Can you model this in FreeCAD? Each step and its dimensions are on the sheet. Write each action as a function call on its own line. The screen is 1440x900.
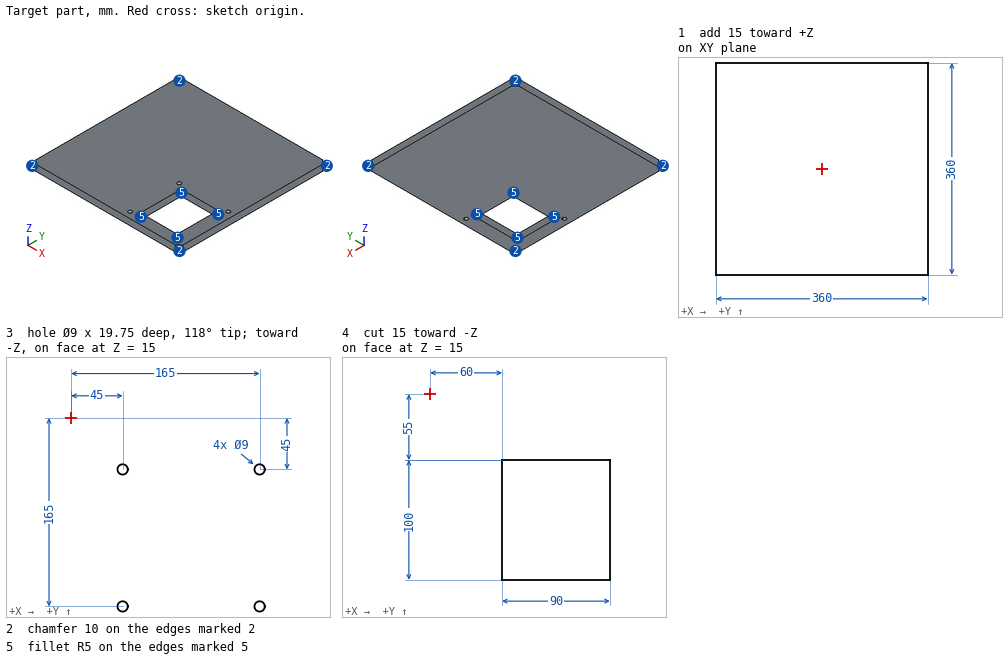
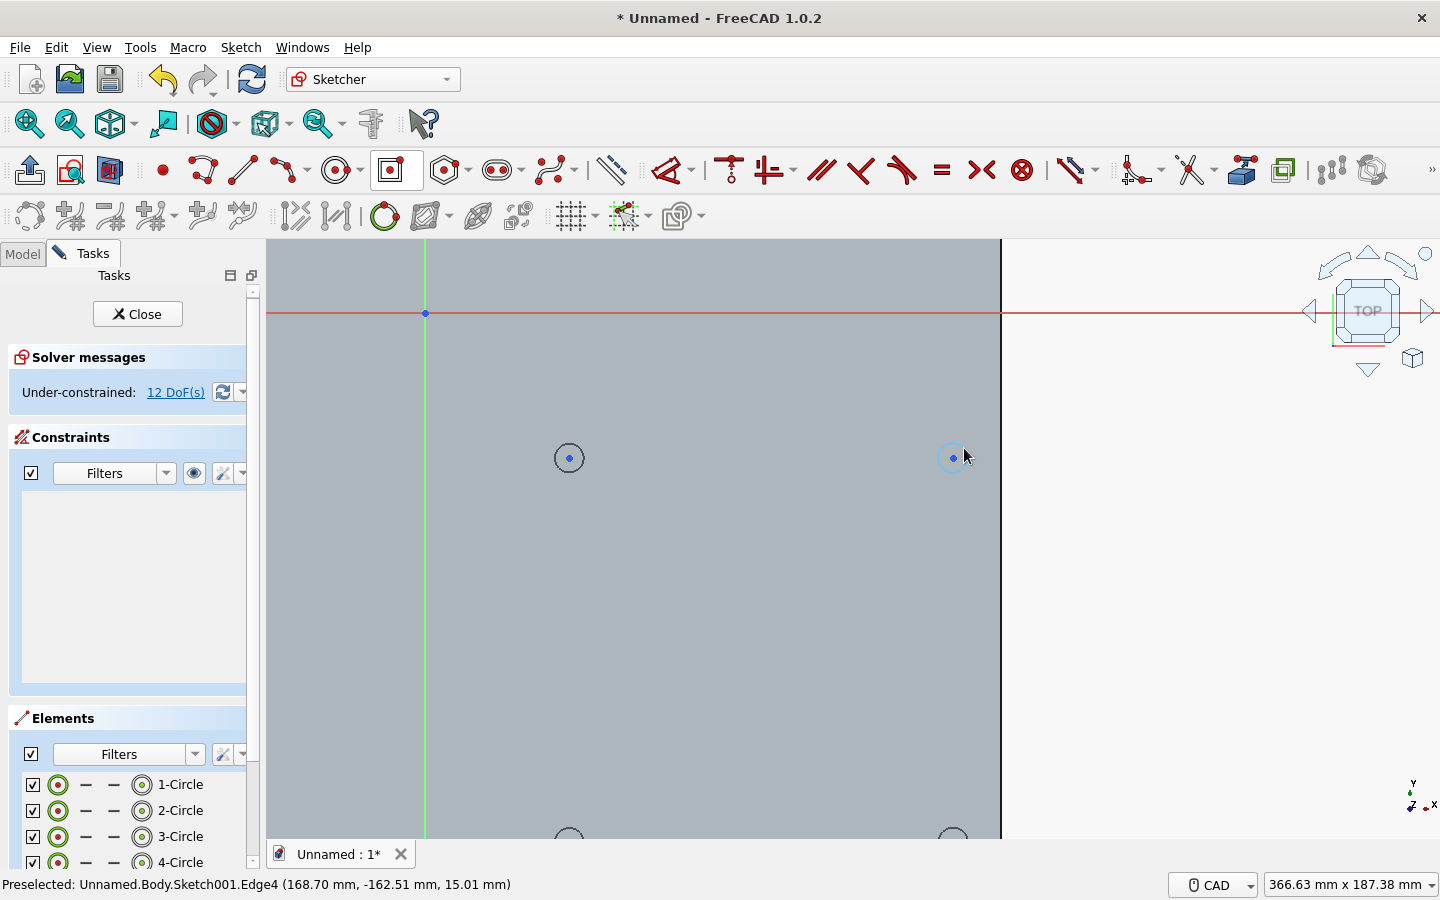
click(964, 448)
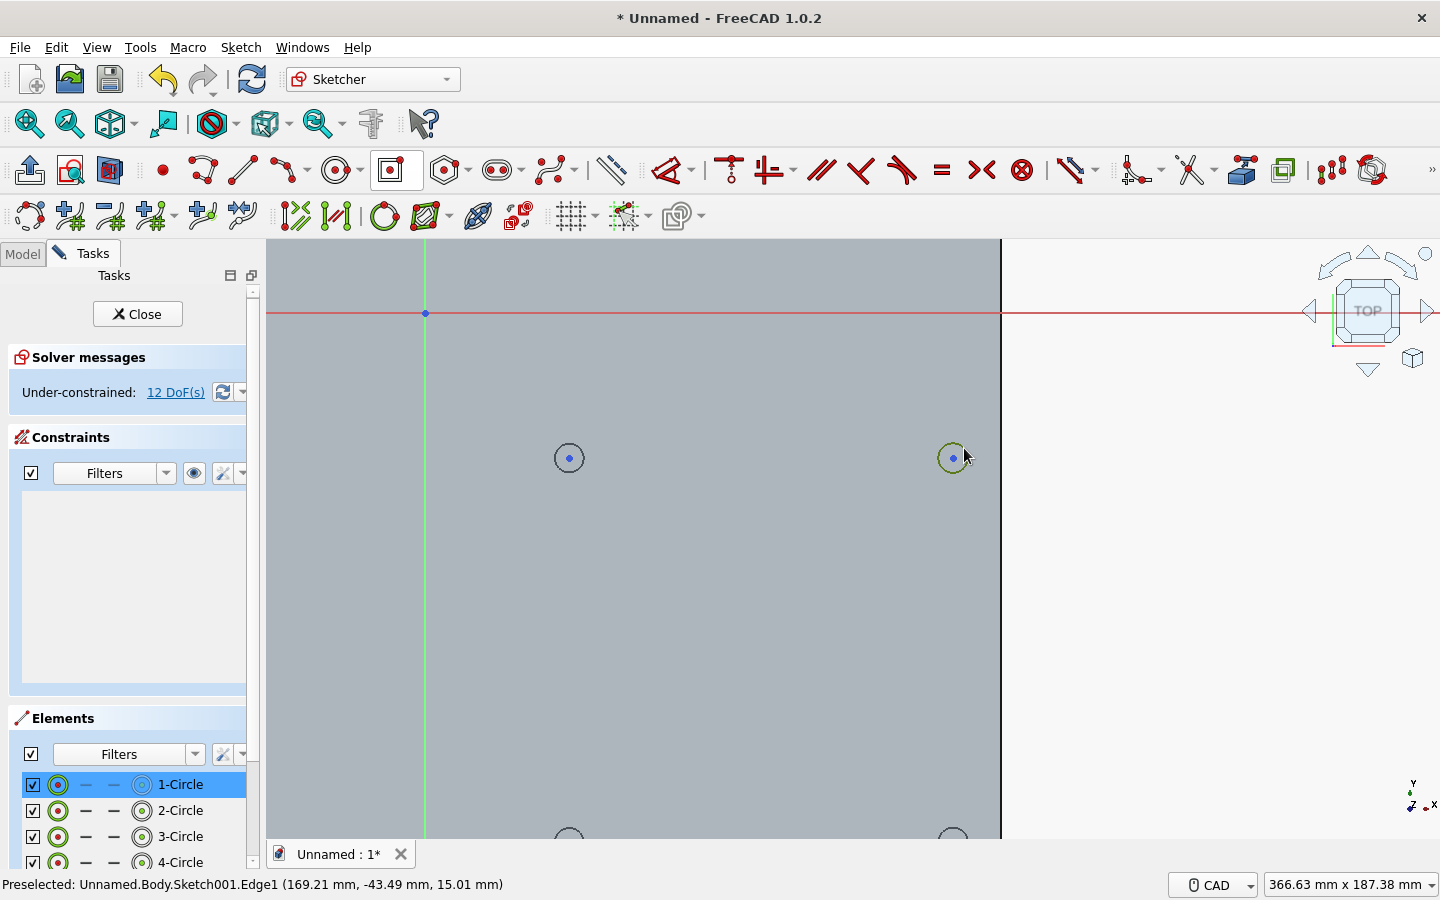
click(579, 448)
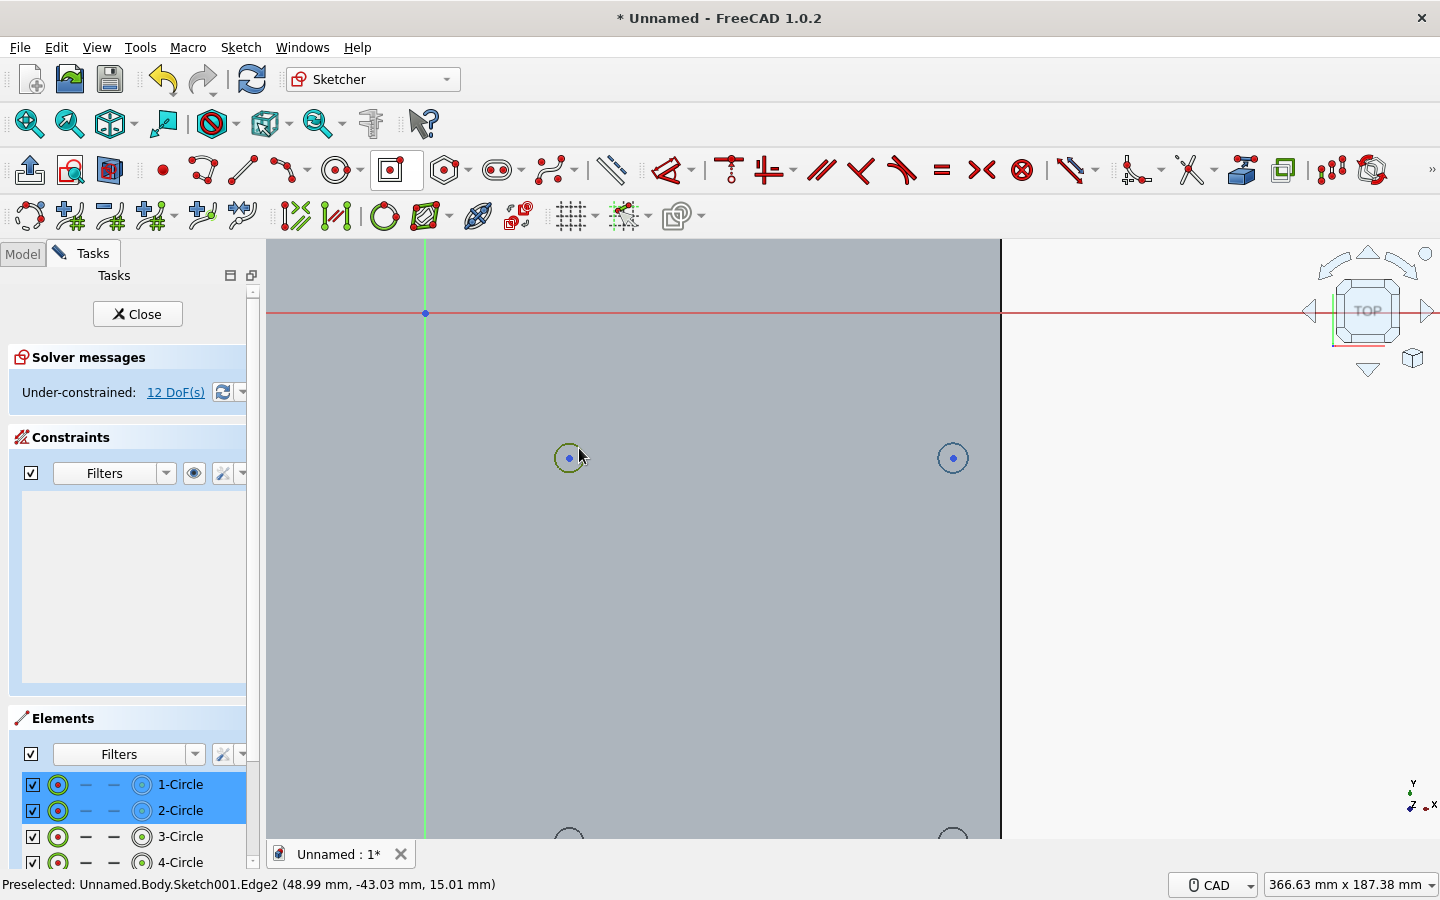
scroll(964, 446, down, 2)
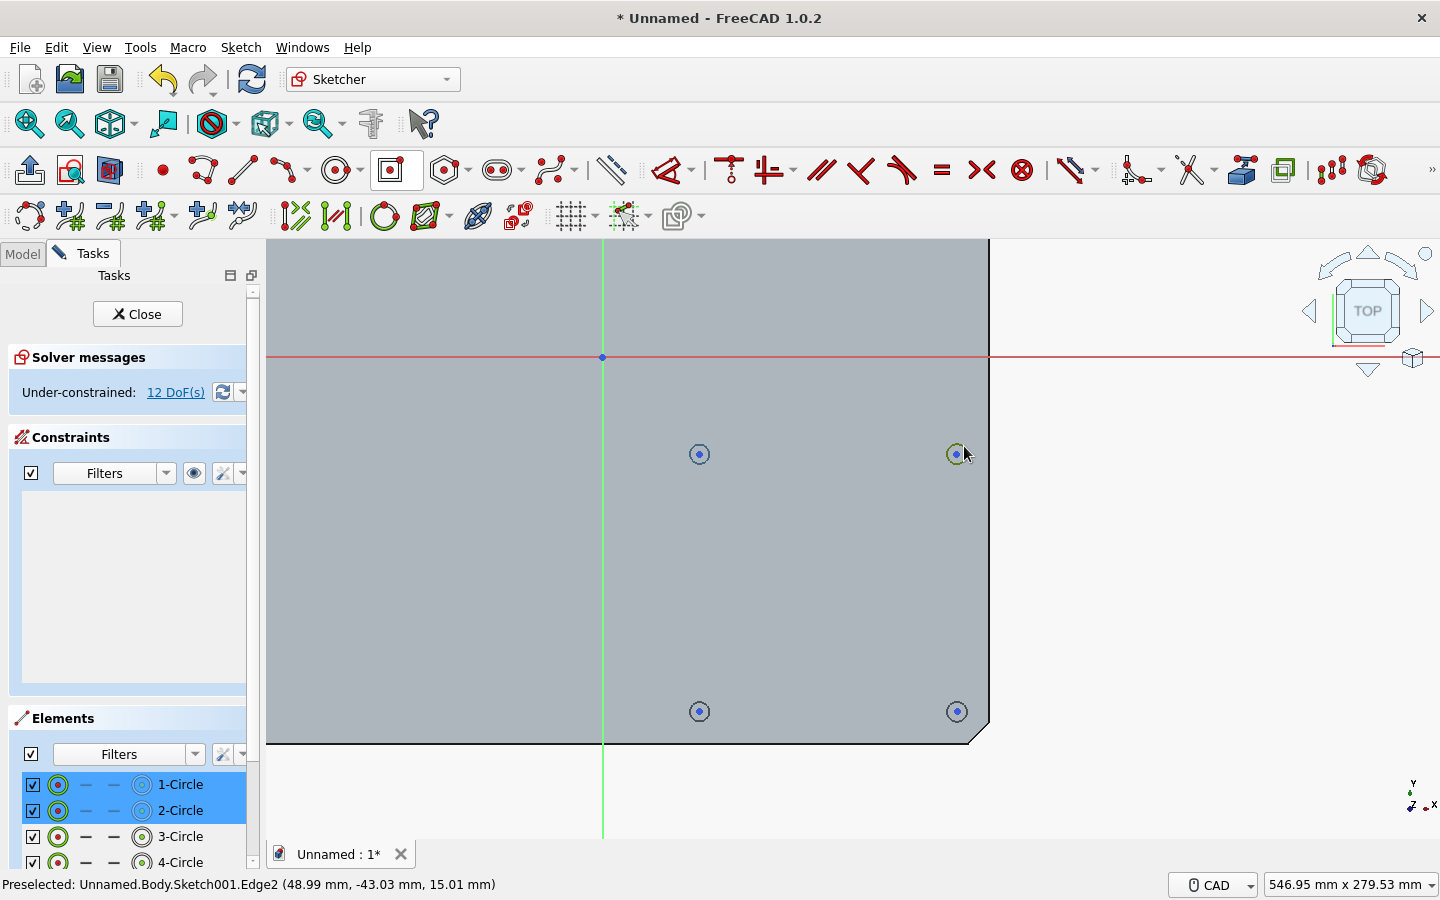
scroll(706, 705, up, 2)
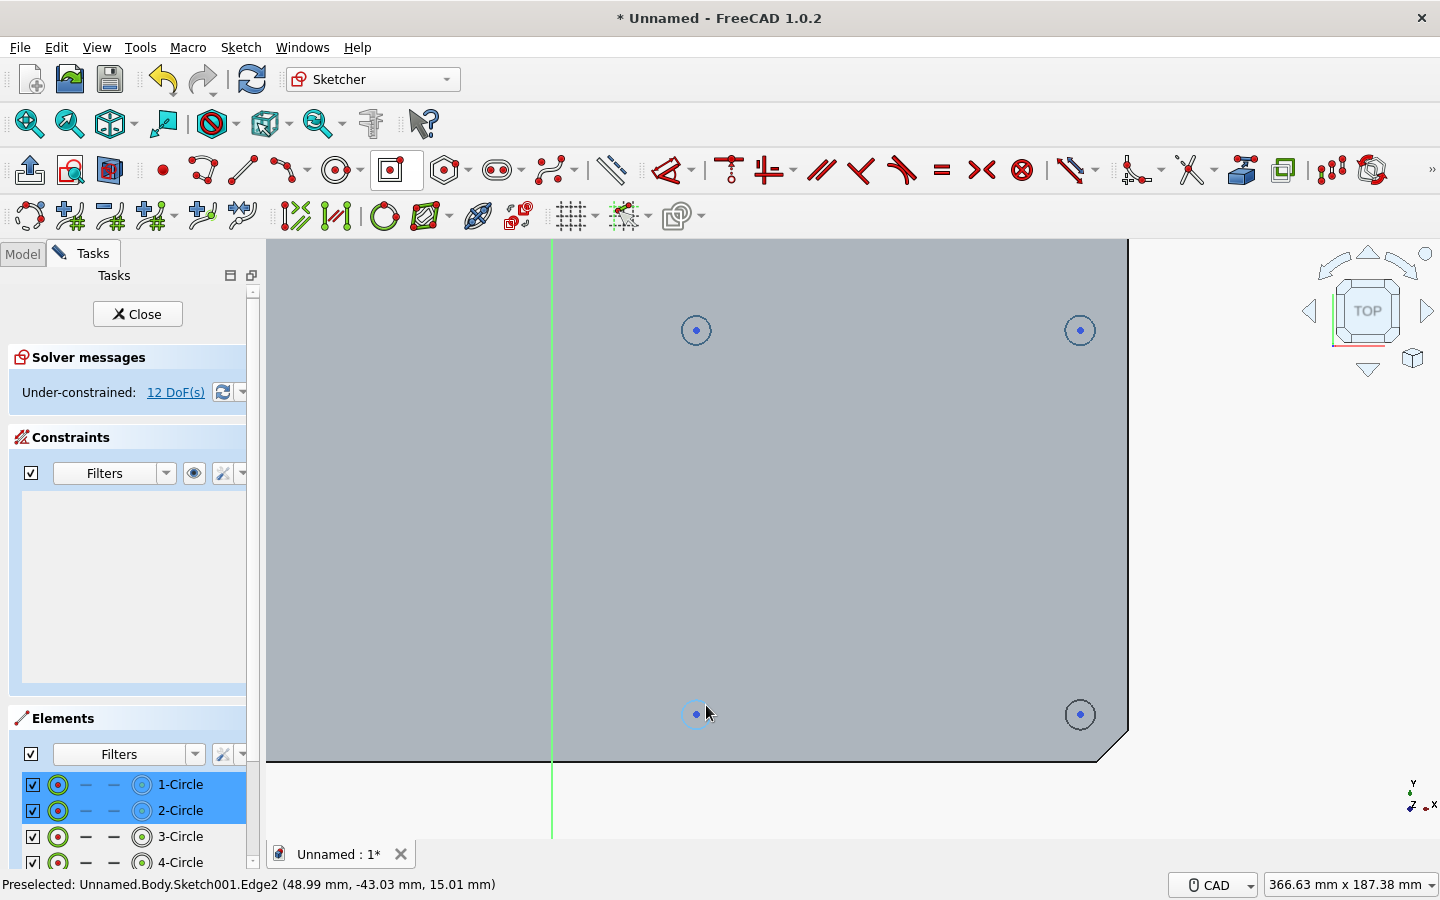
click(706, 705)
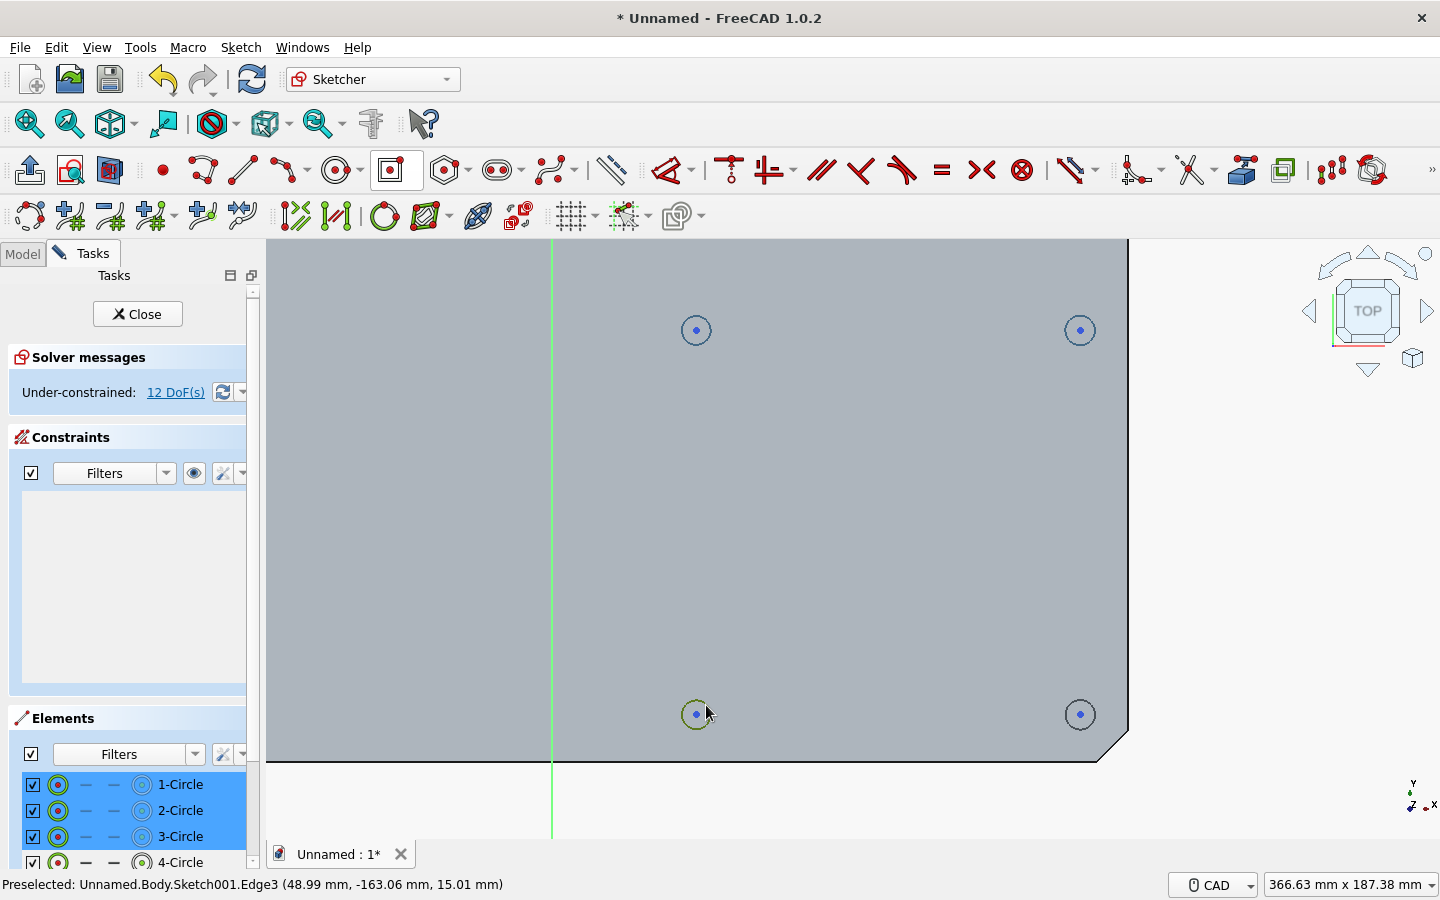
click(1091, 704)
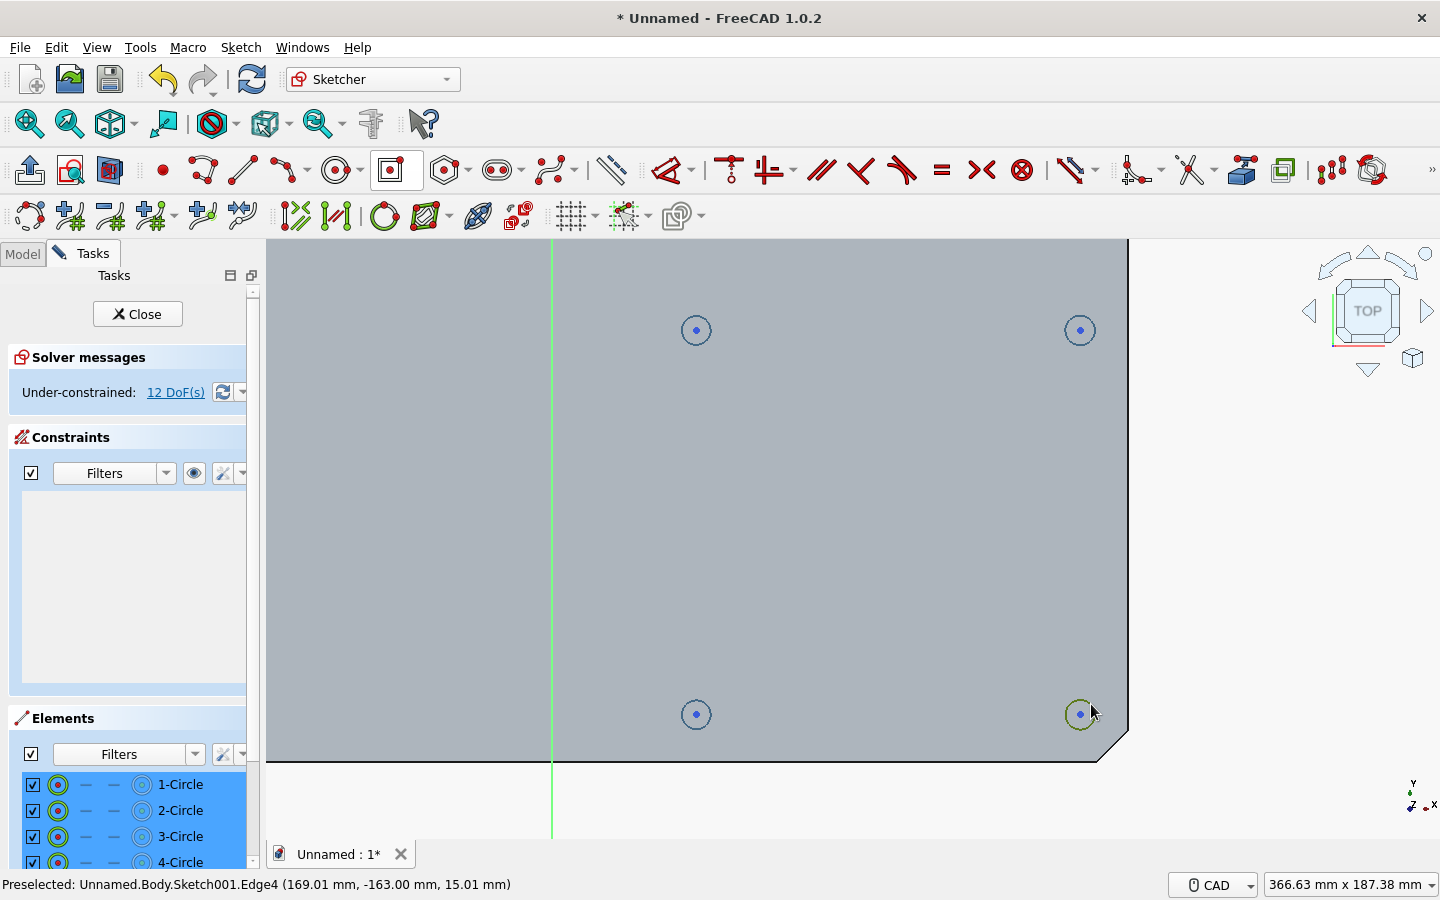
key(e)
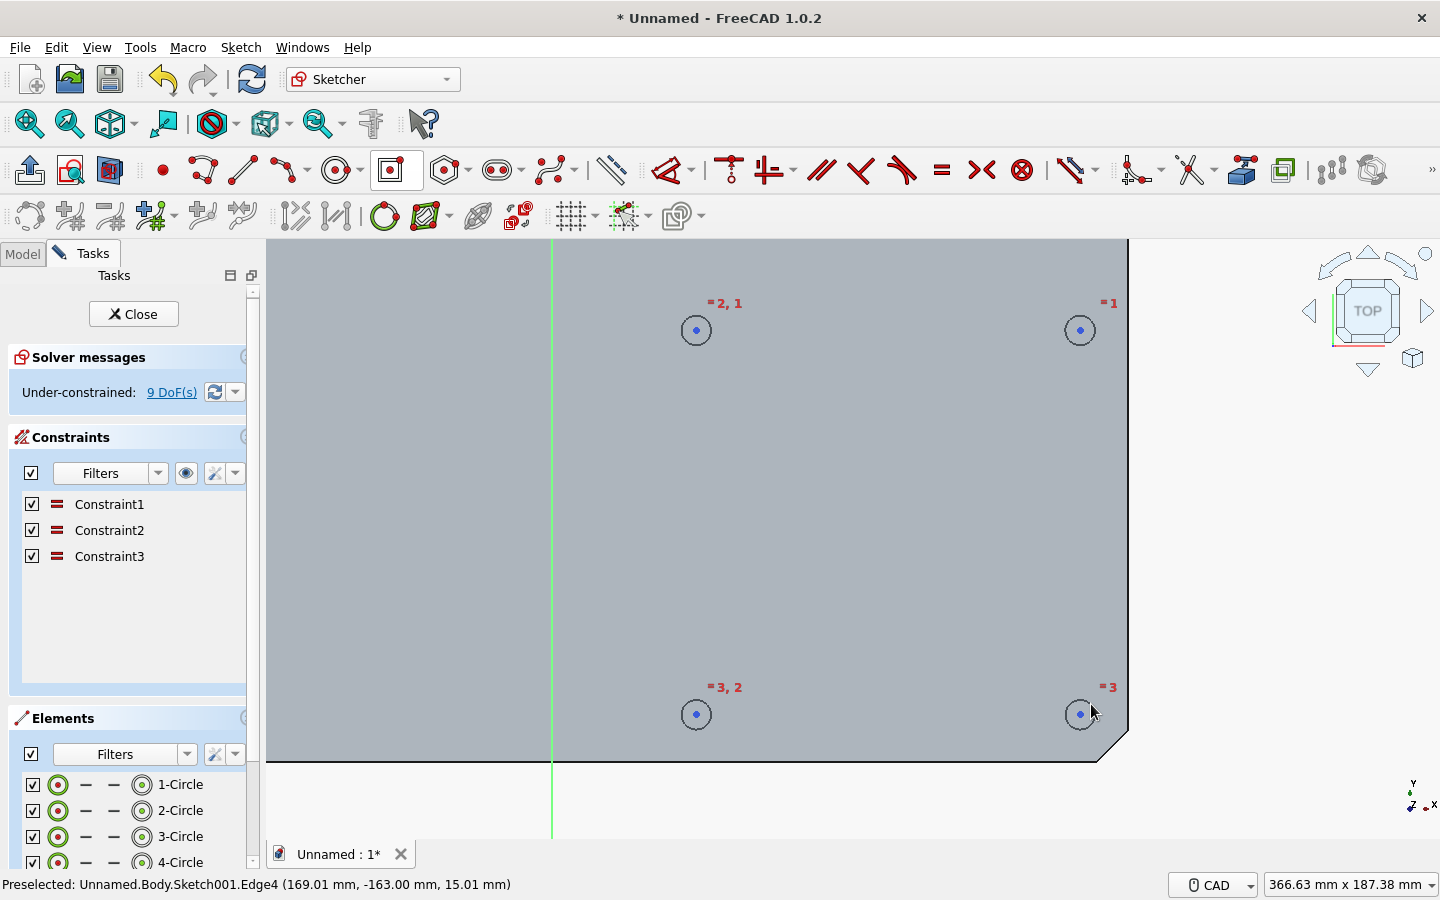
click(1080, 330)